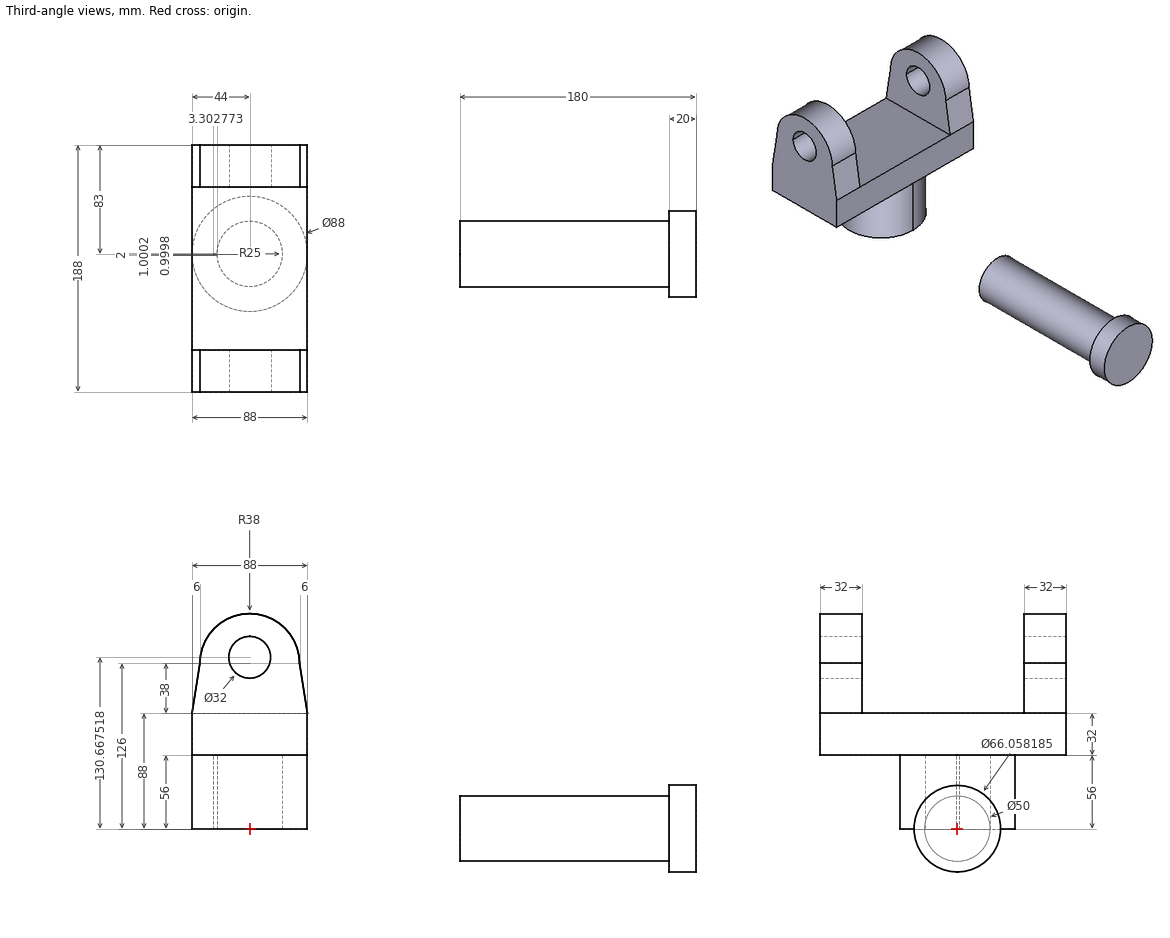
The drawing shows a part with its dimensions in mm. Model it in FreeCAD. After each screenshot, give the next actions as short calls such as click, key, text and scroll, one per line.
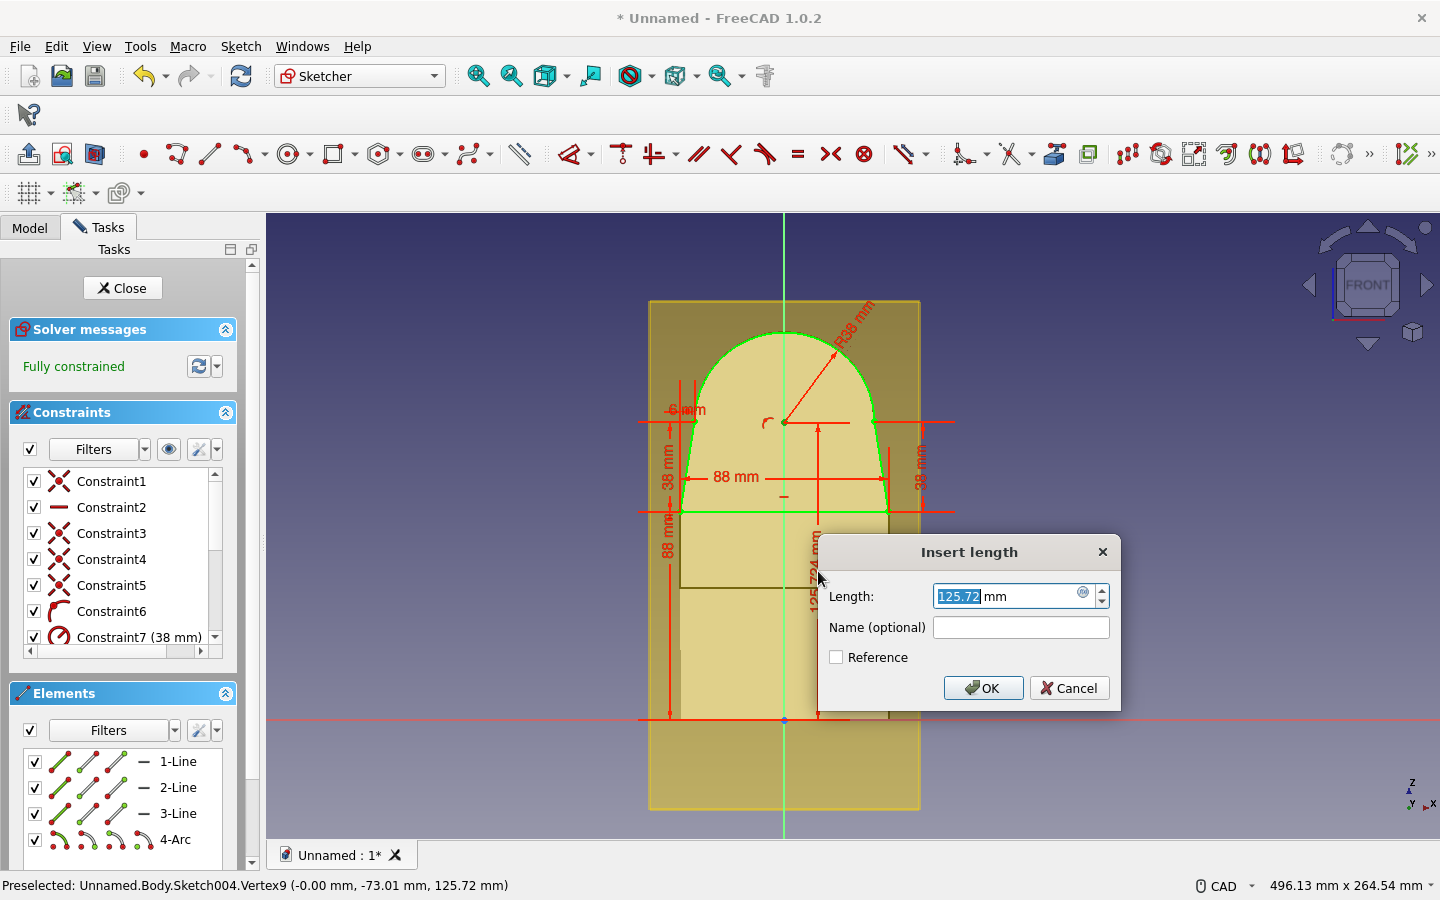
text(126)
key(Return)
key(Escape)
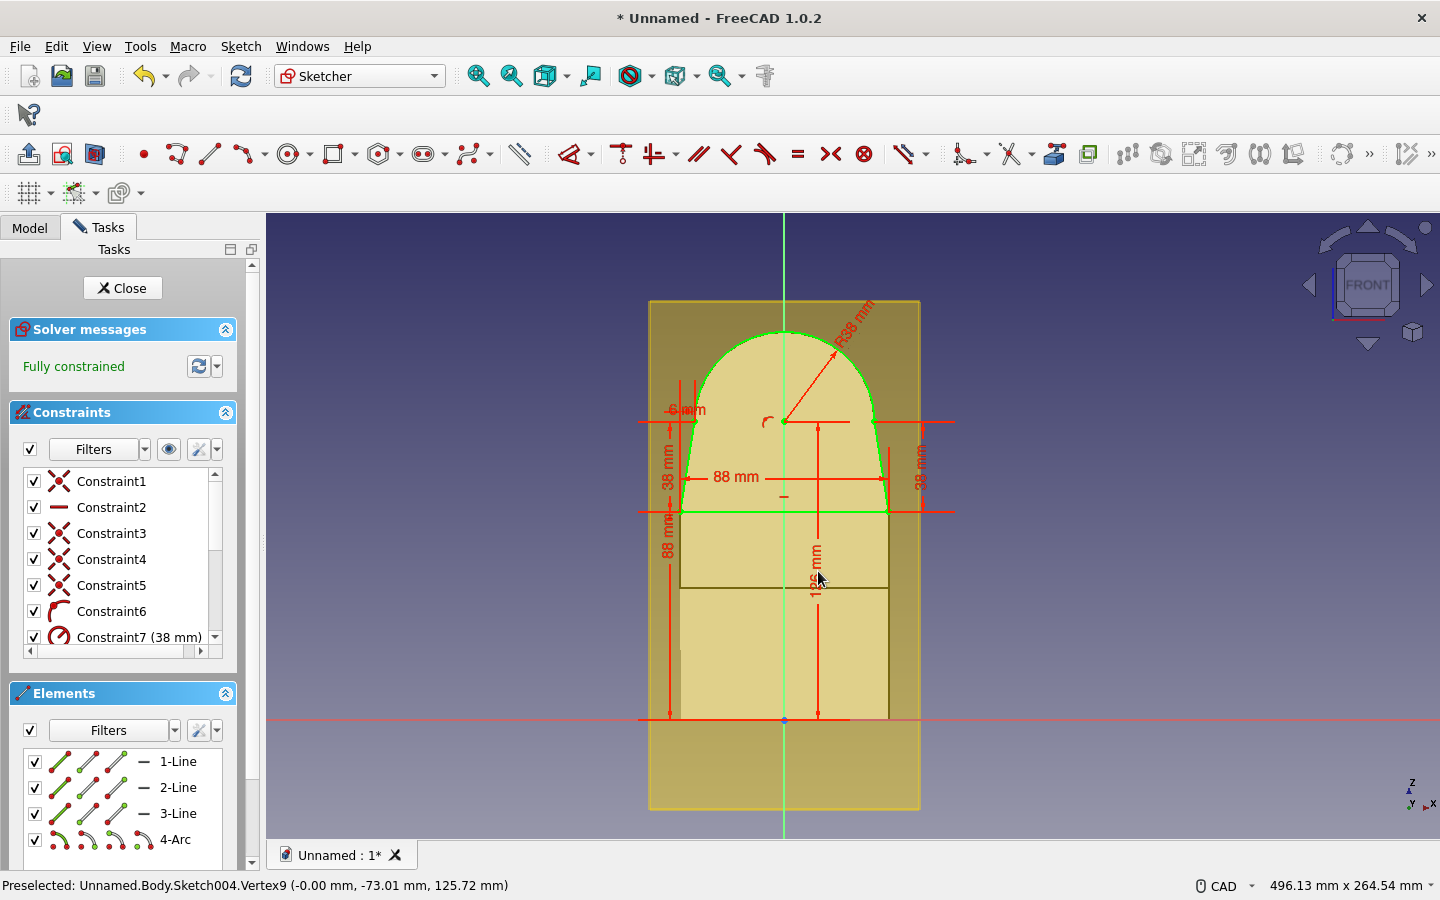
click(123, 288)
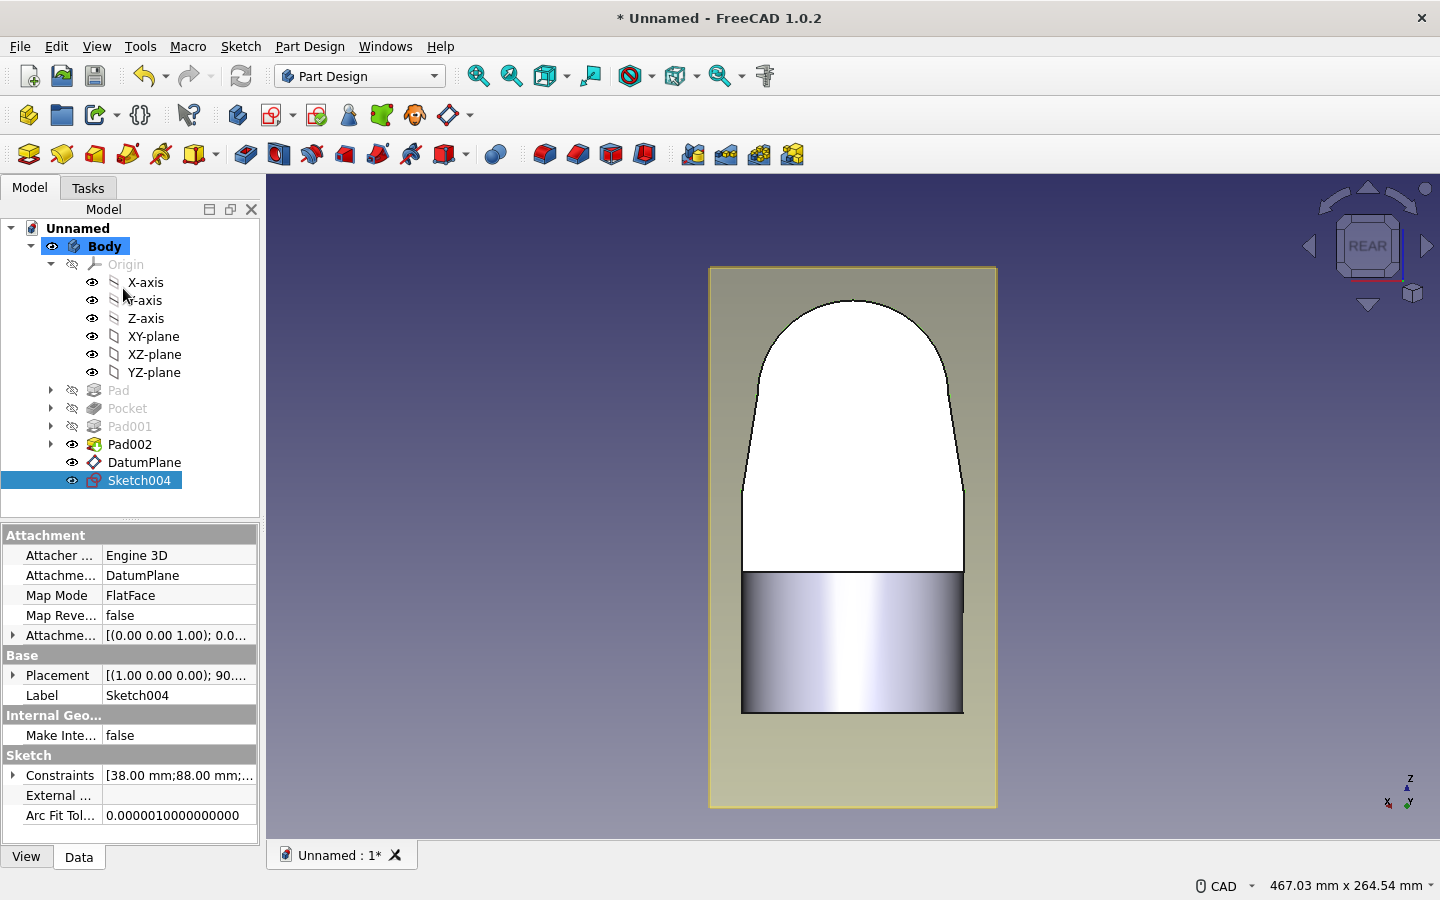
click(29, 154)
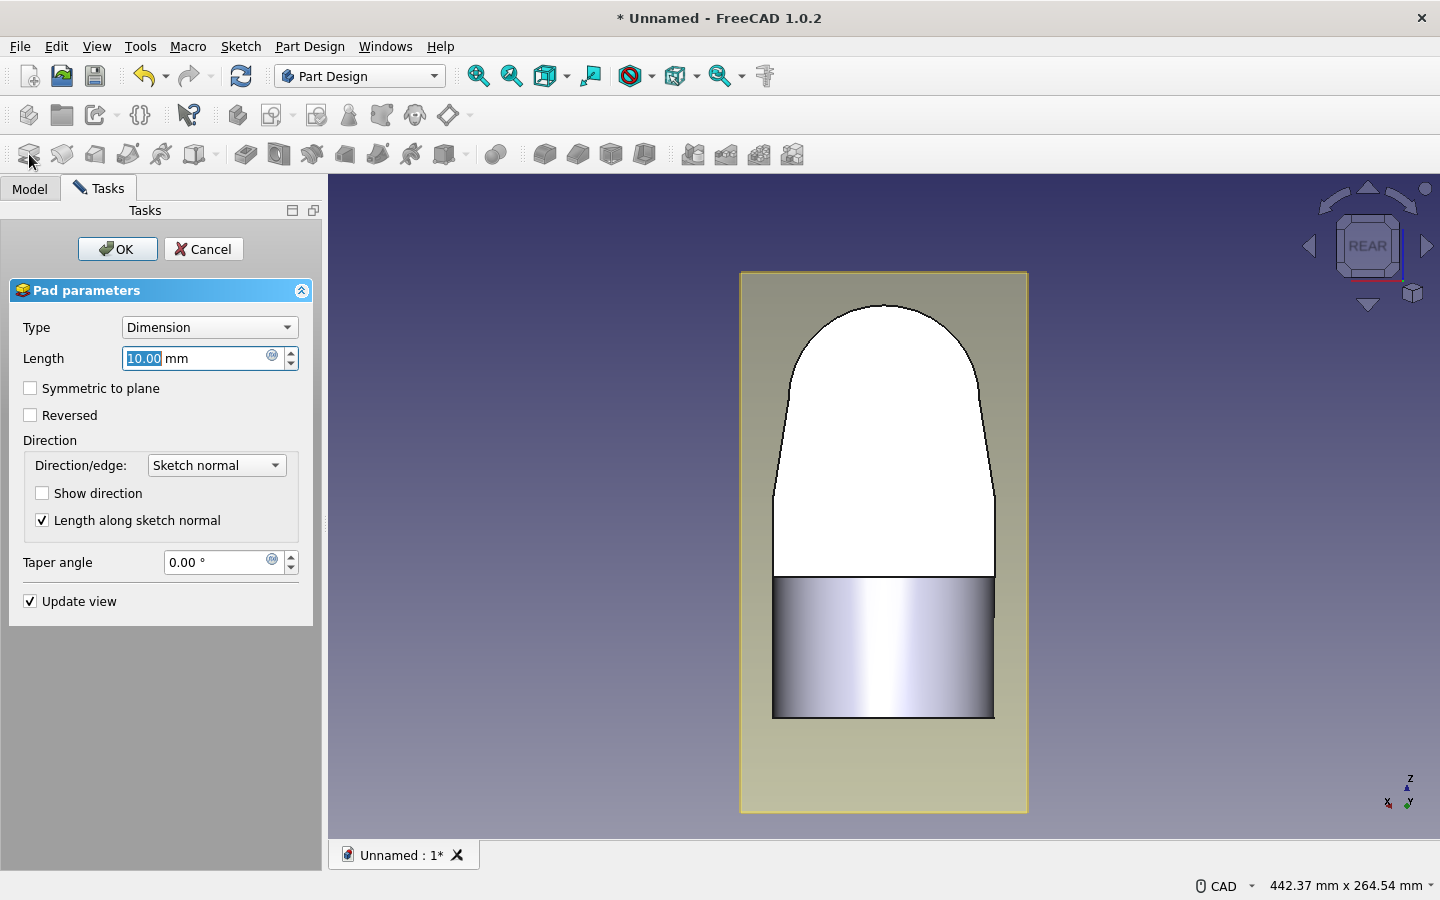
text(32)
key(Tab)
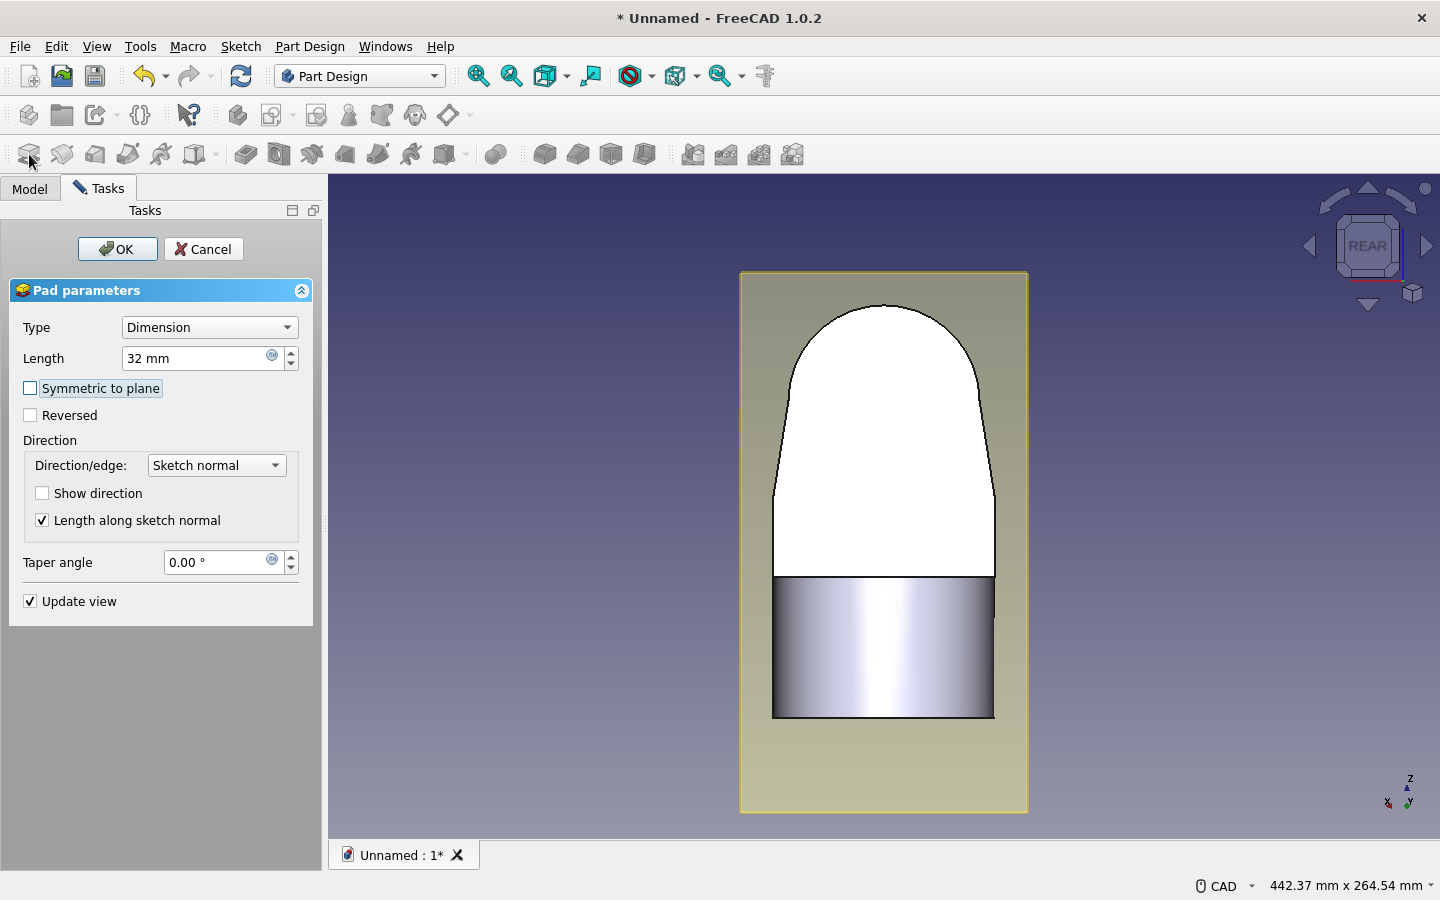
click(118, 249)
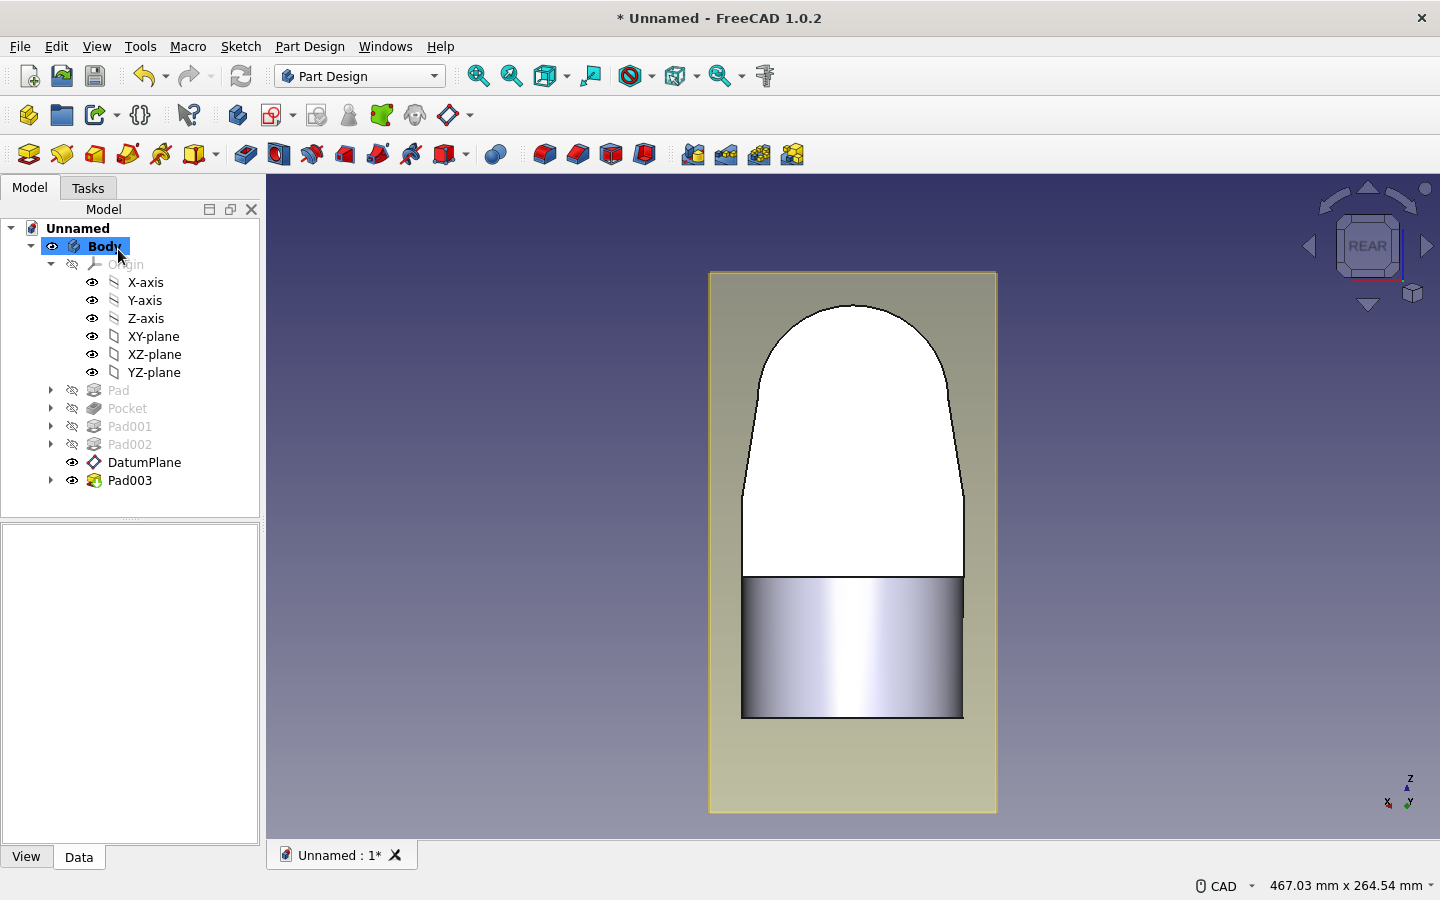
click(117, 462)
key(space)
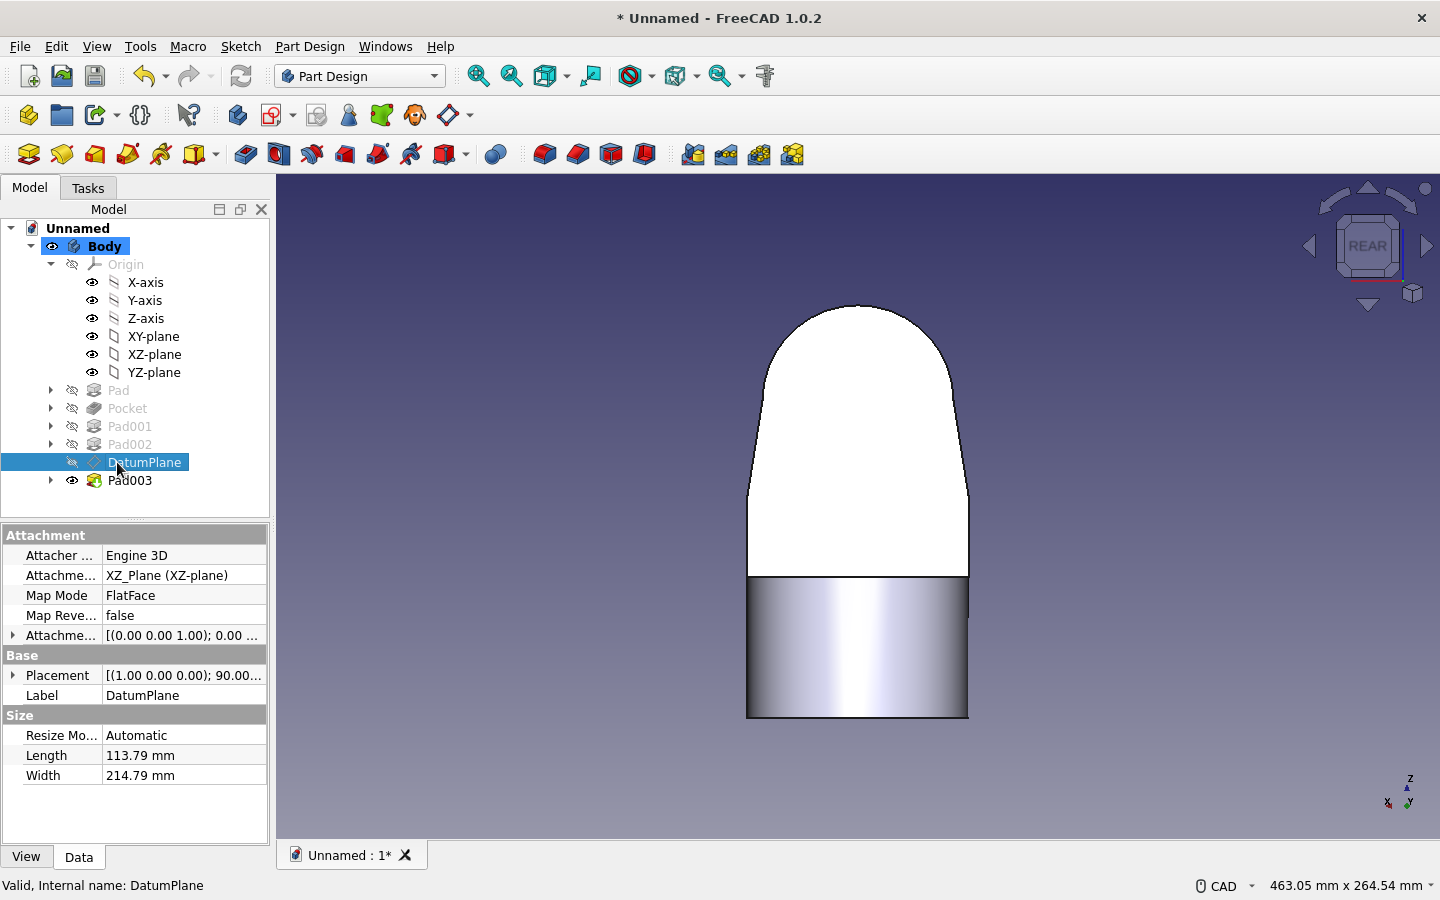
click(858, 440)